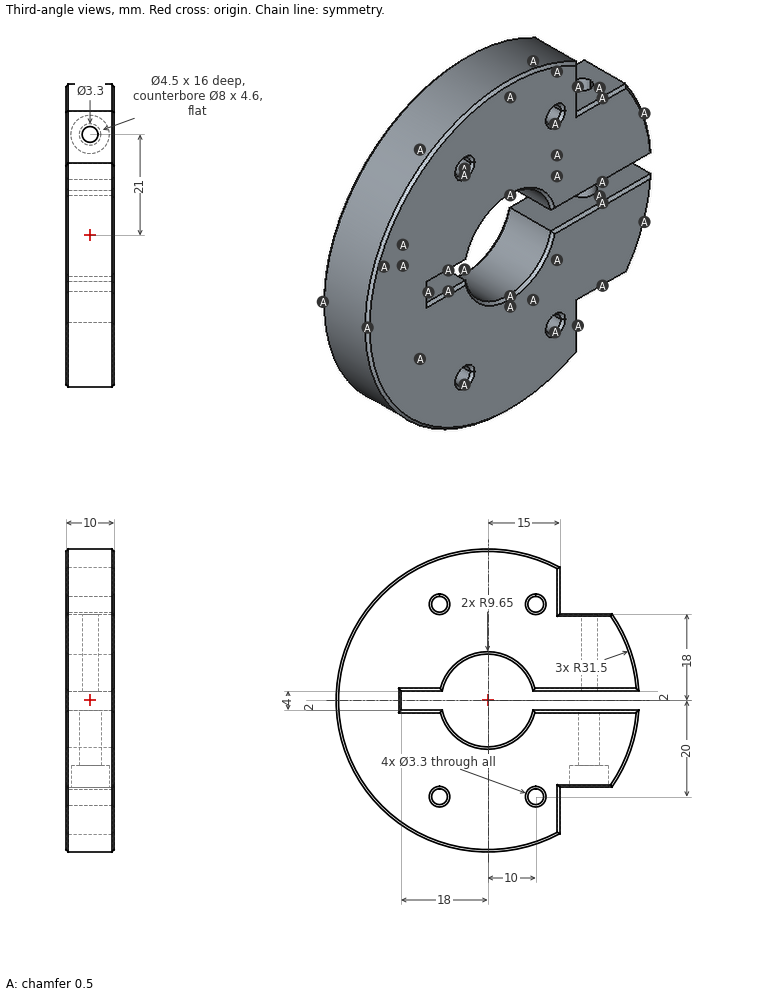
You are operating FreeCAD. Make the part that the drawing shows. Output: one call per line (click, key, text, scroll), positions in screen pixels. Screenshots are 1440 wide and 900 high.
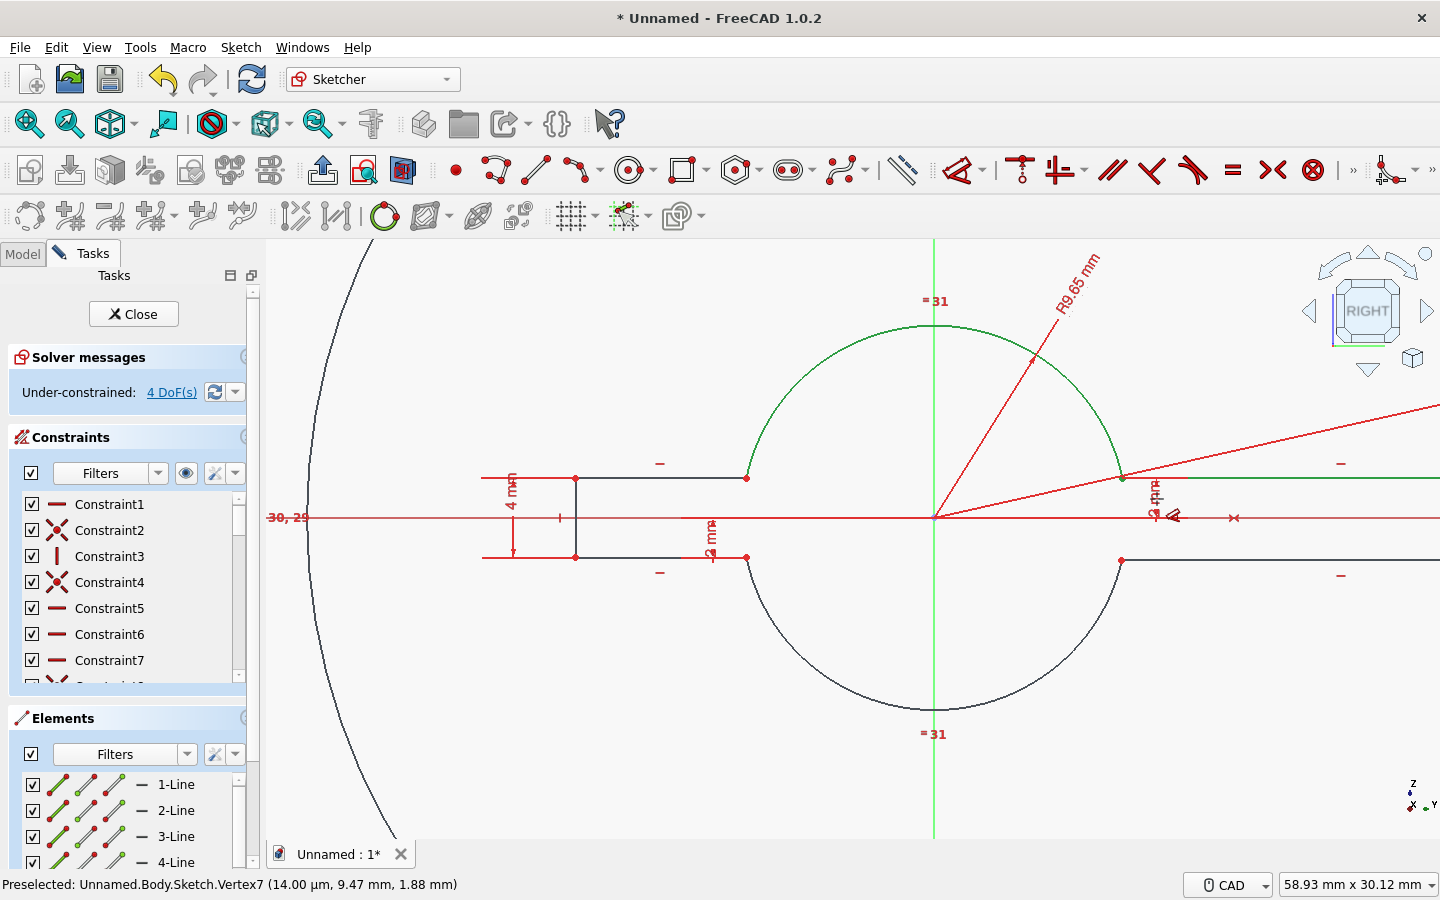
scroll(698, 551, down, 5)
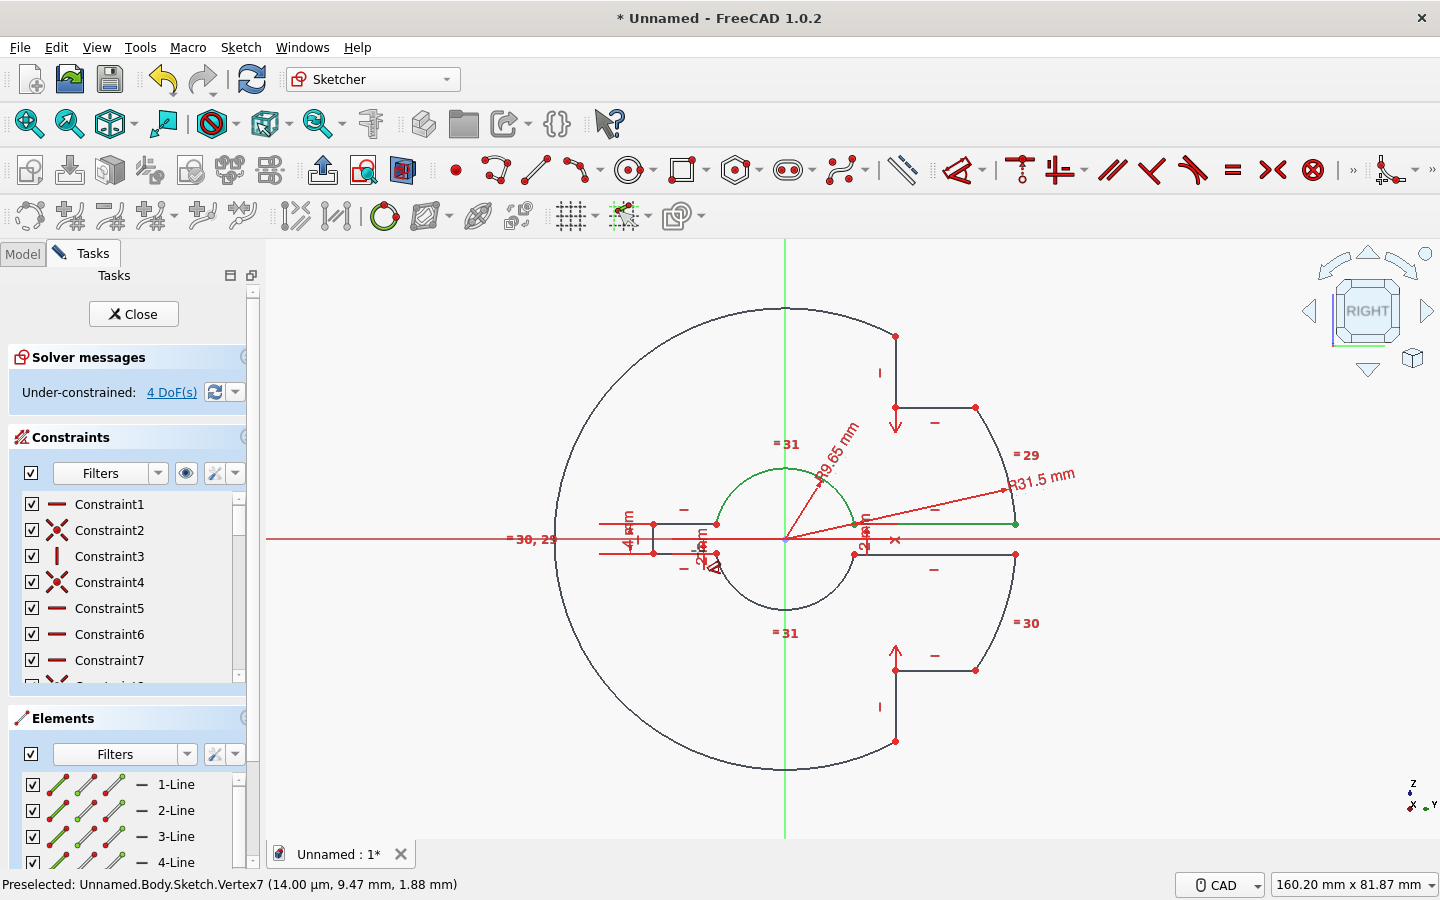
scroll(1016, 555, up, 5)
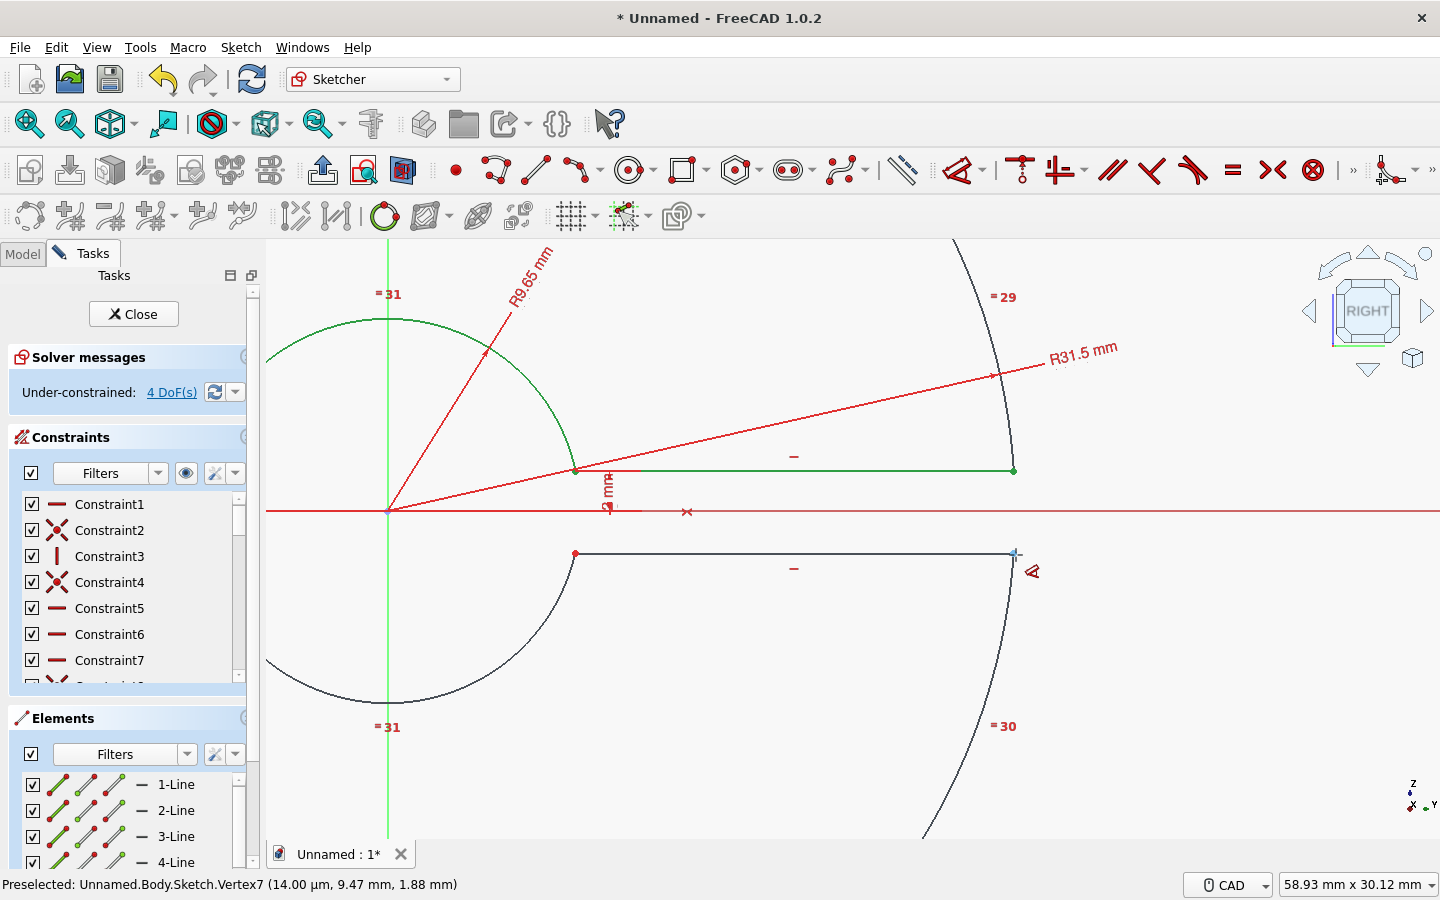
click(1014, 554)
click(1048, 532)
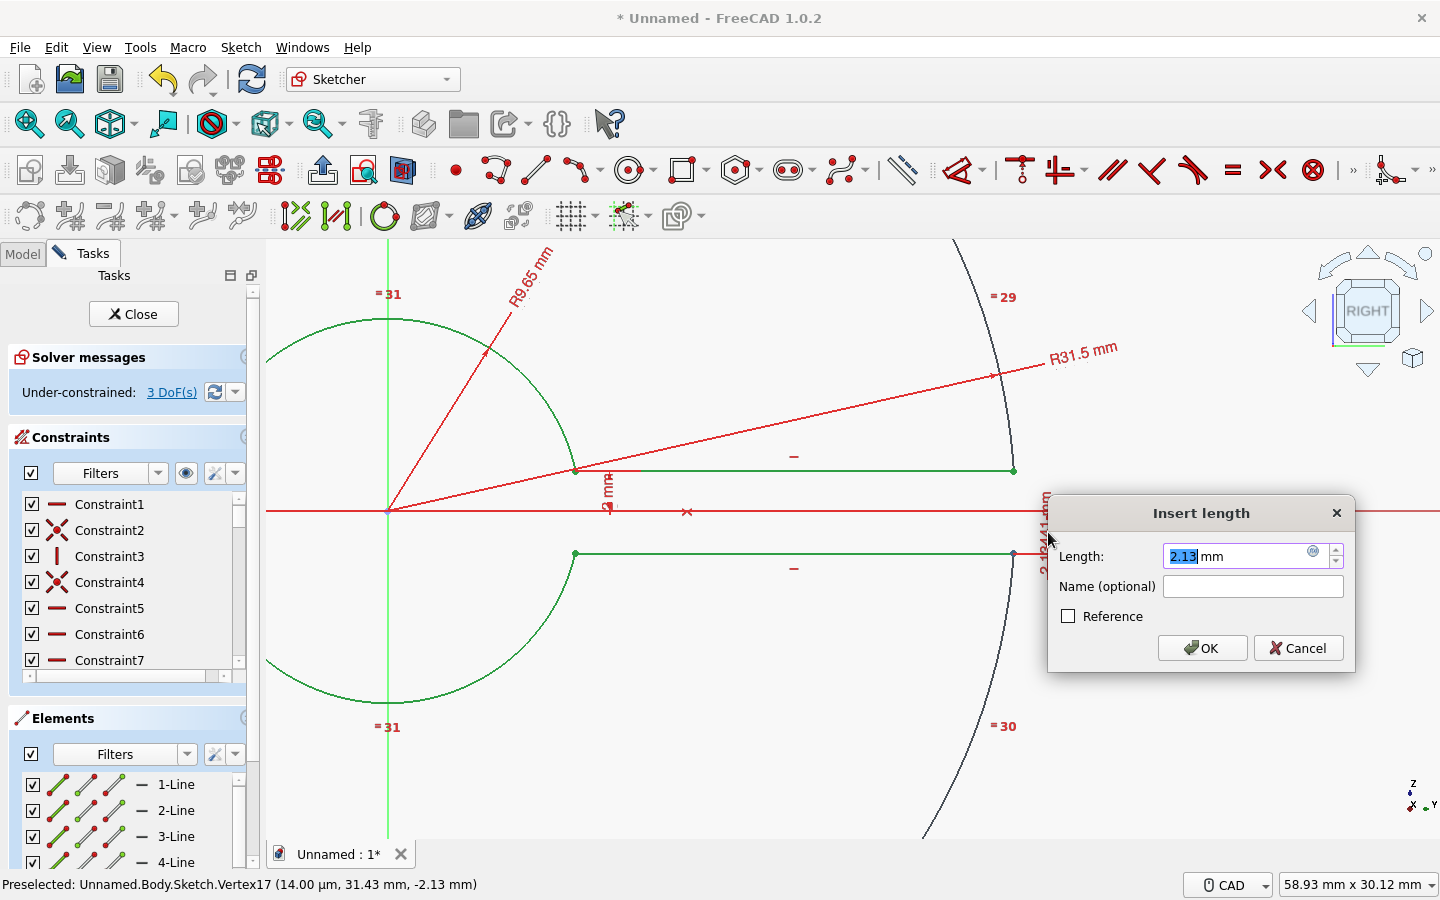
text(2)
key(Return)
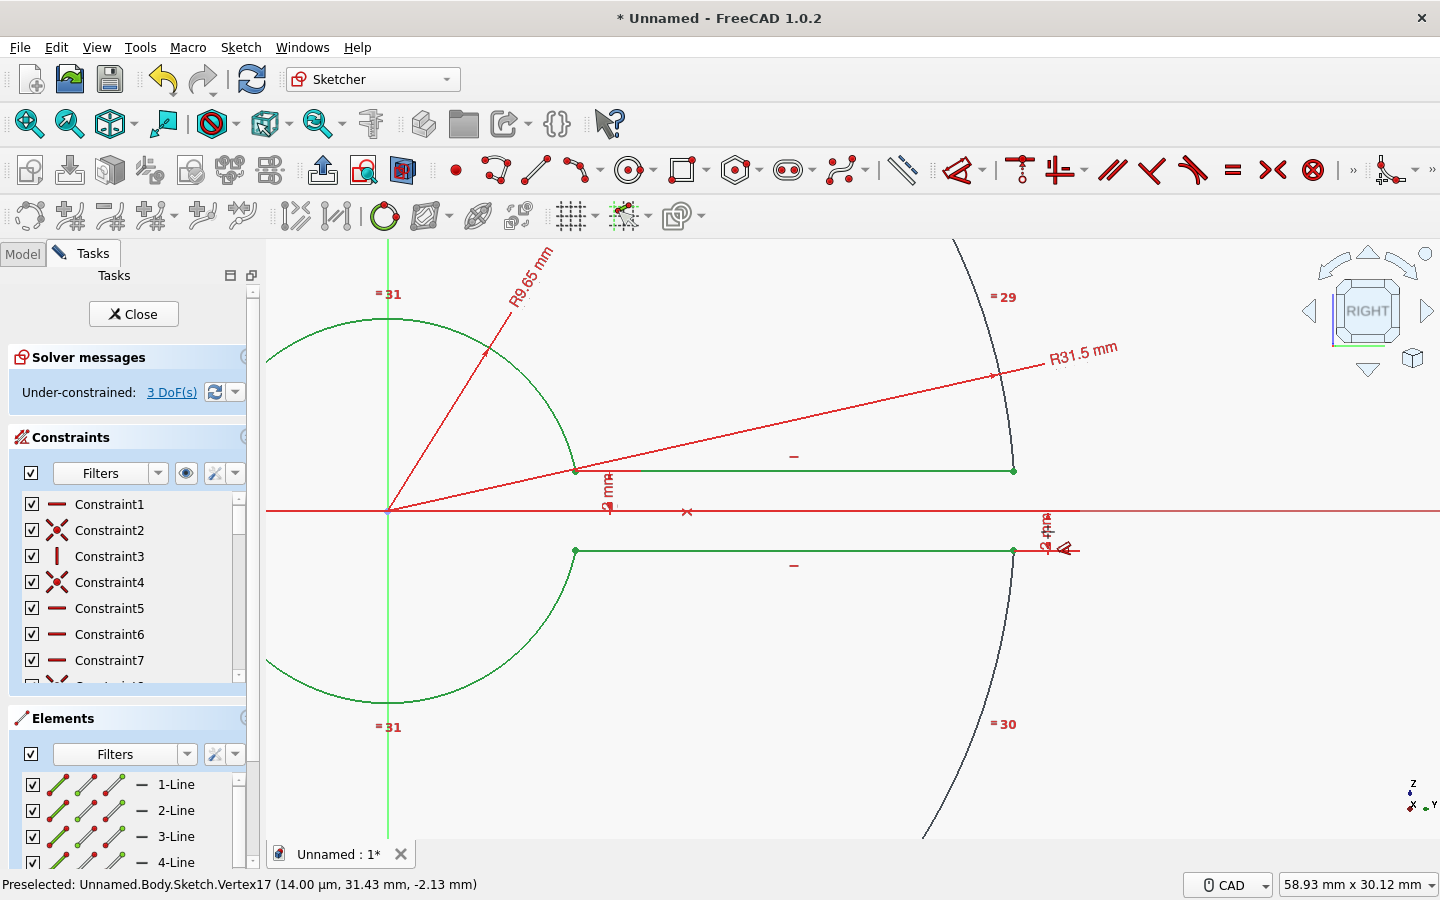
scroll(1016, 555, down, 5)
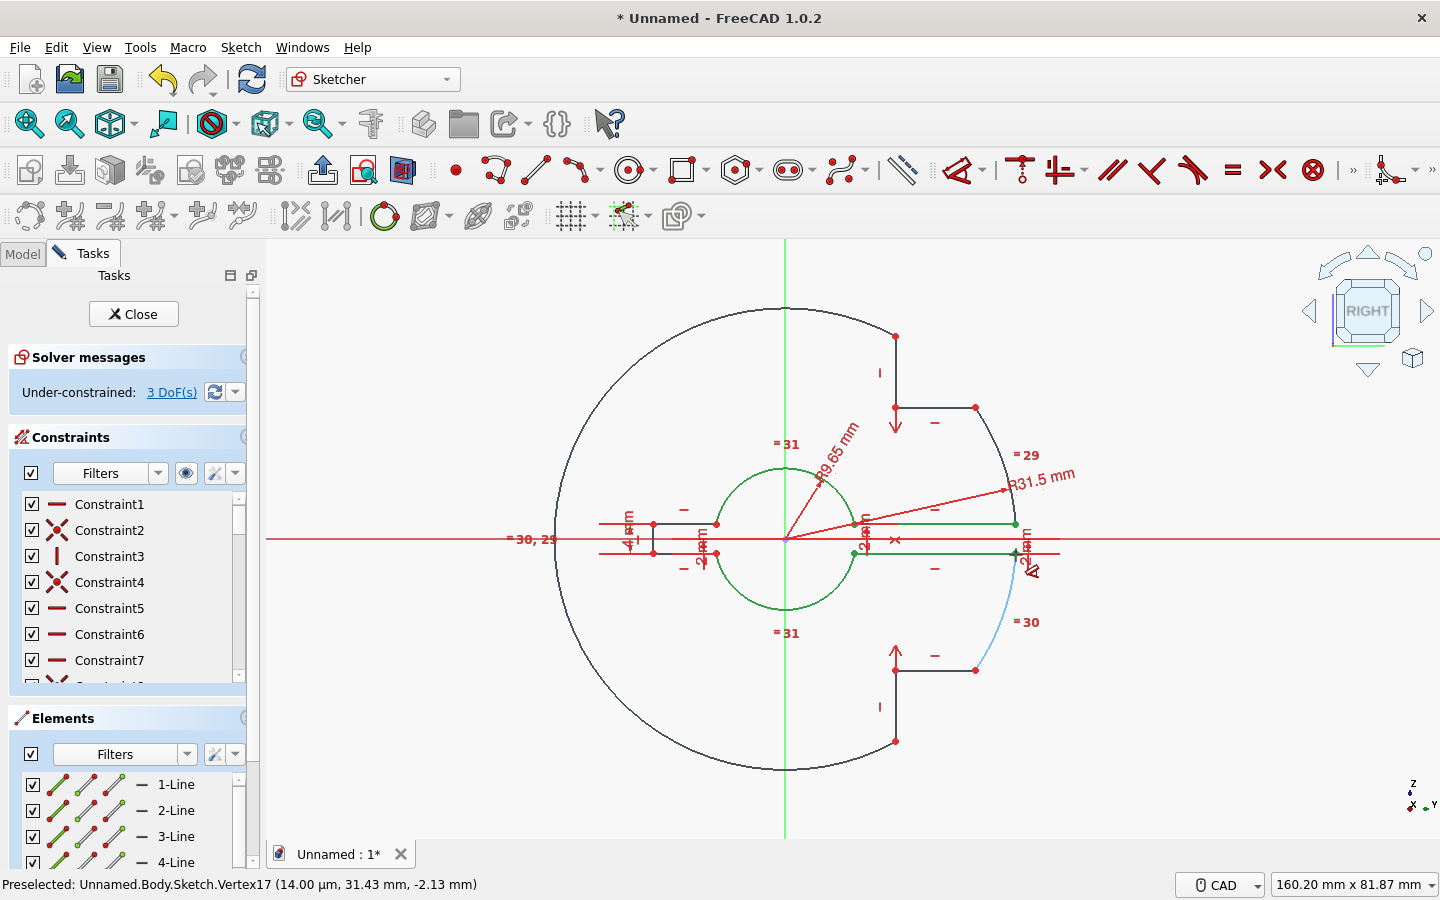
click(653, 554)
click(689, 588)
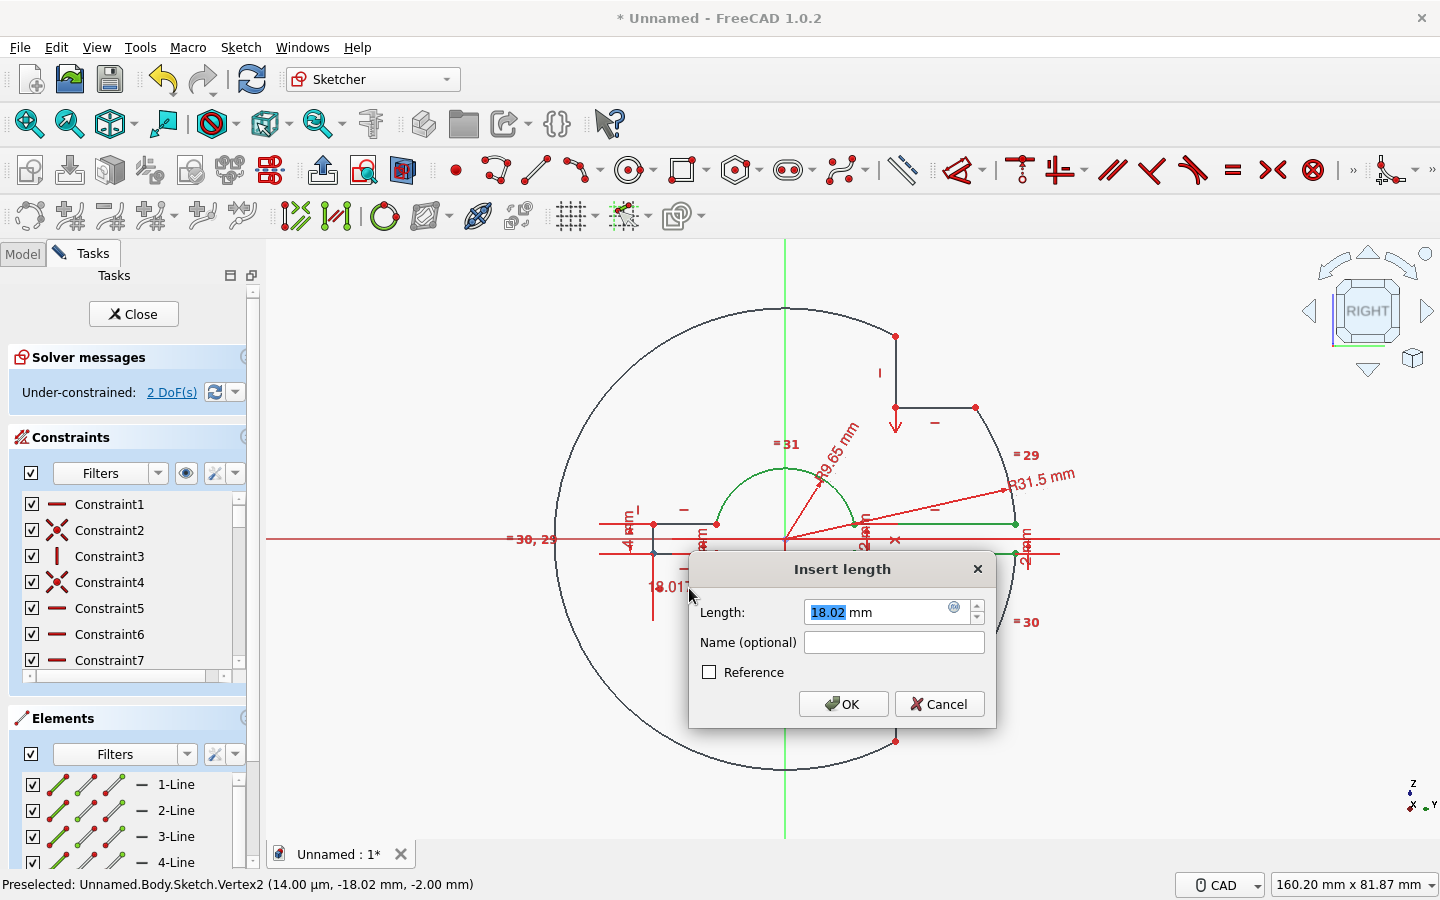
text(18)
key(Return)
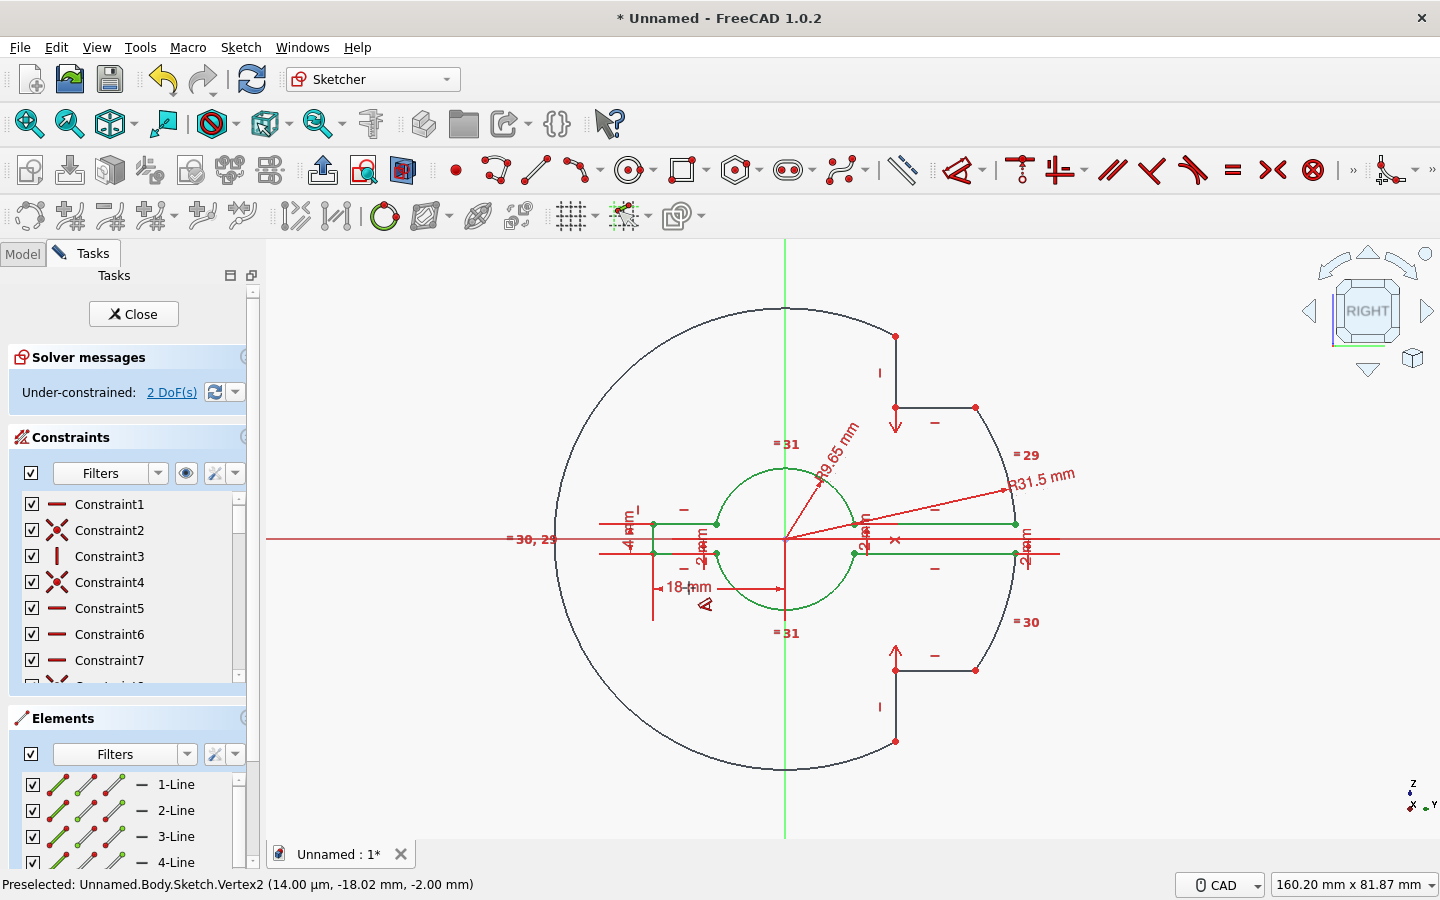
click(975, 408)
click(1009, 427)